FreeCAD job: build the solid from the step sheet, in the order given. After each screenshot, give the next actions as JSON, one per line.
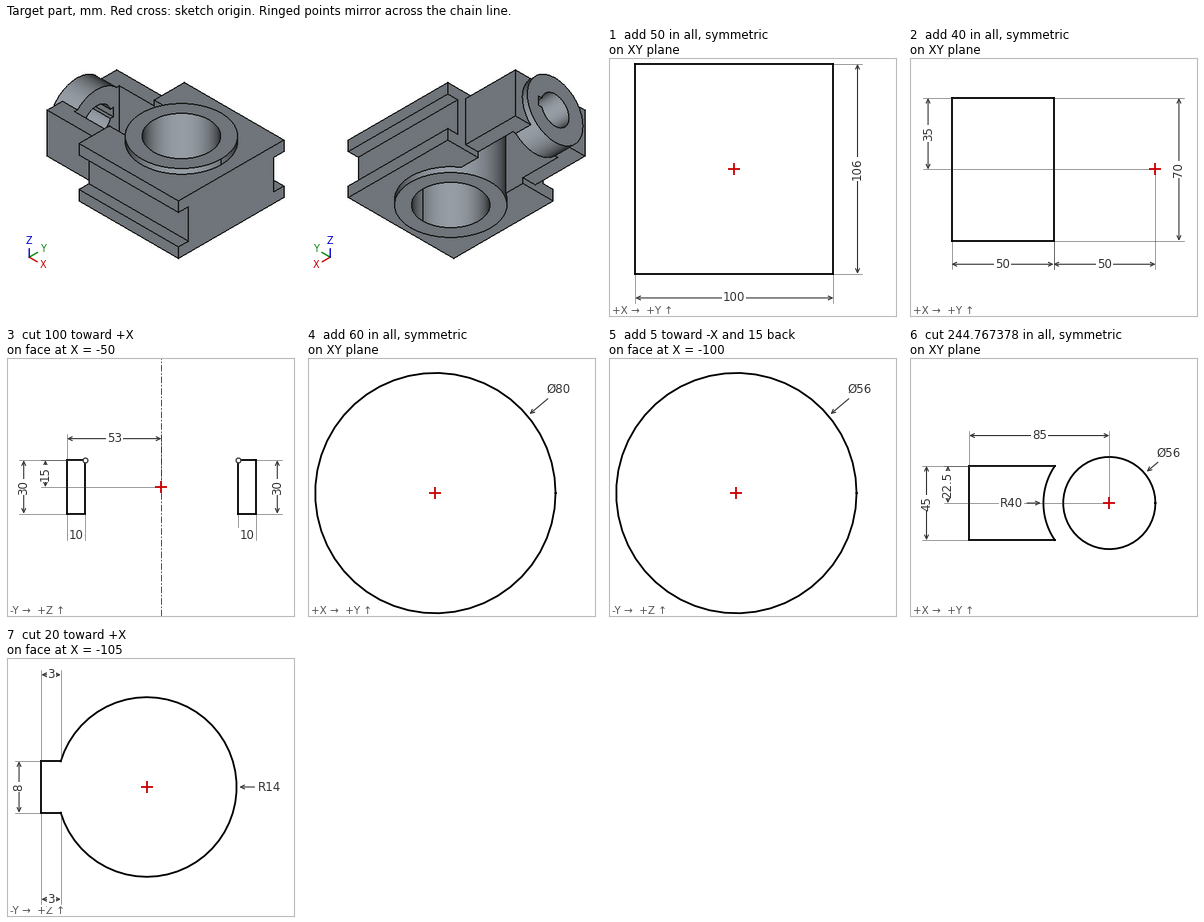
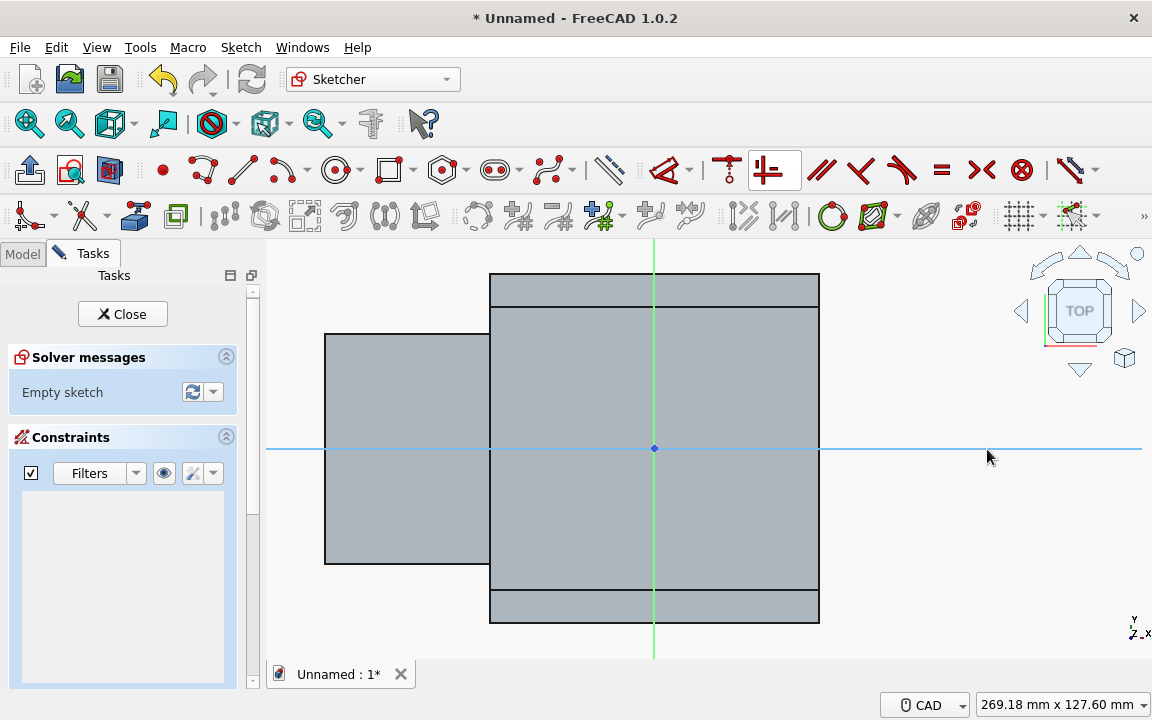
{"action": "left_click", "coordinate": [336, 170]}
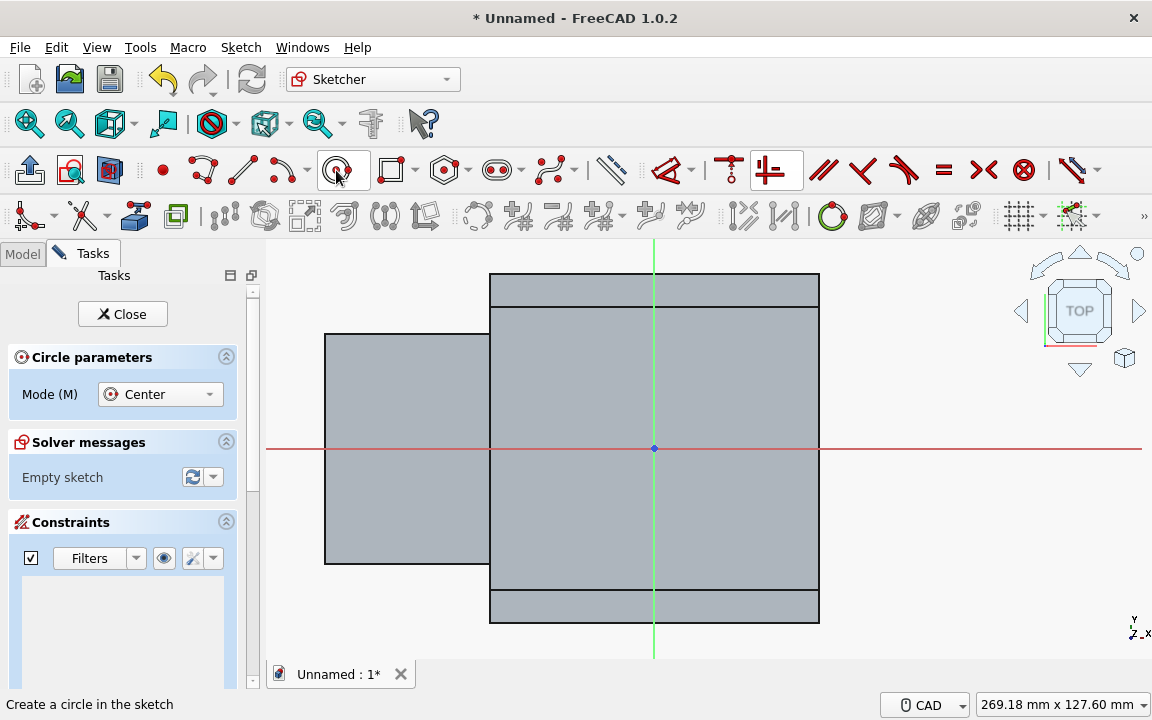
{"action": "left_click", "coordinate": [654, 449]}
{"action": "mouse_move", "coordinate": [747, 356]}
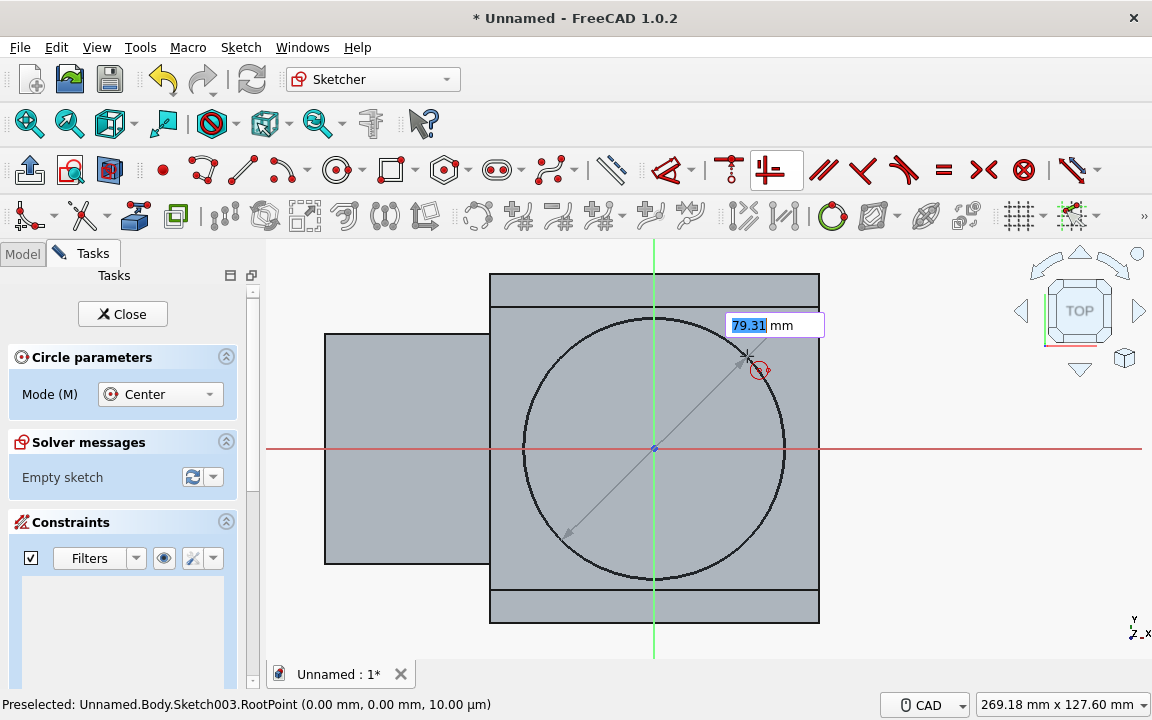
{"action": "type", "text": "80"}
{"action": "key", "text": "Return"}
{"action": "key", "text": "Escape"}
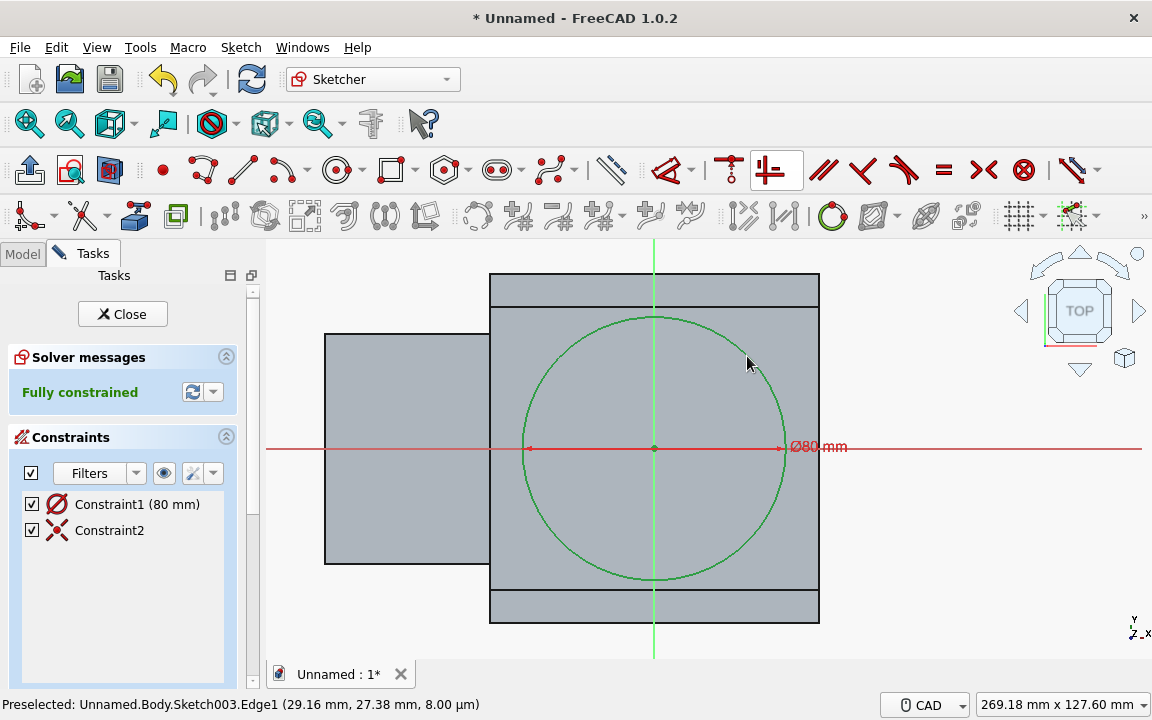
{"action": "left_click", "coordinate": [123, 314]}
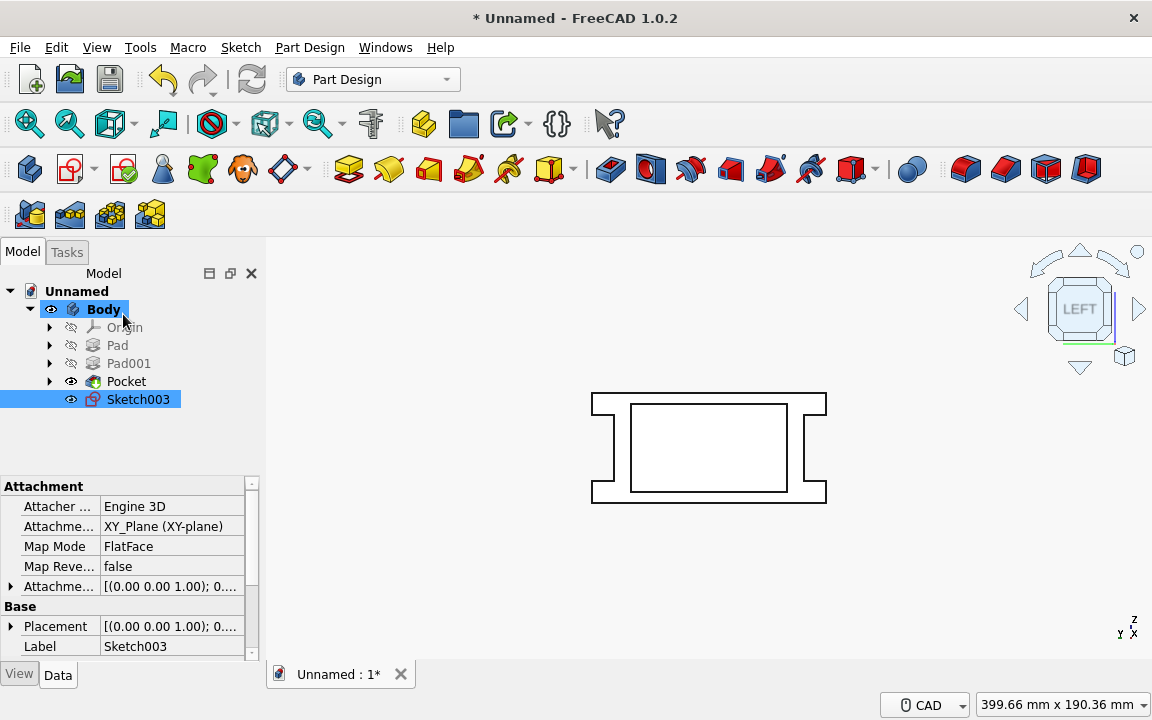
{"action": "left_click", "coordinate": [350, 170]}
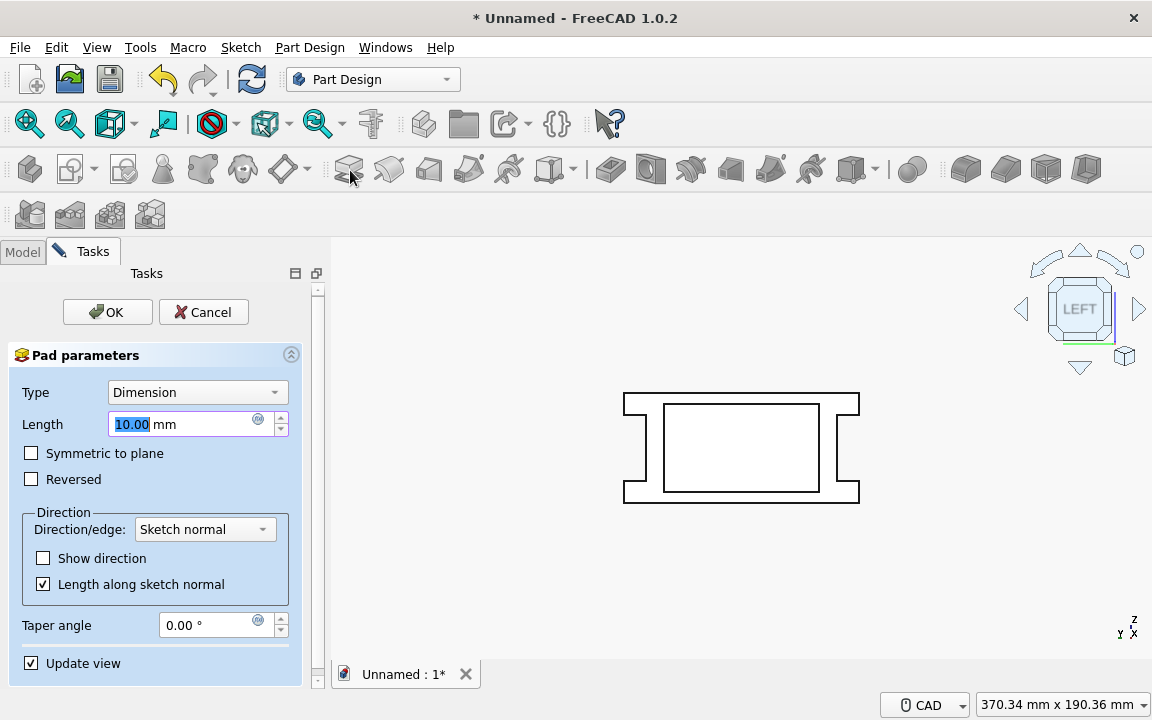
{"action": "type", "text": "60"}
{"action": "key", "text": "Tab"}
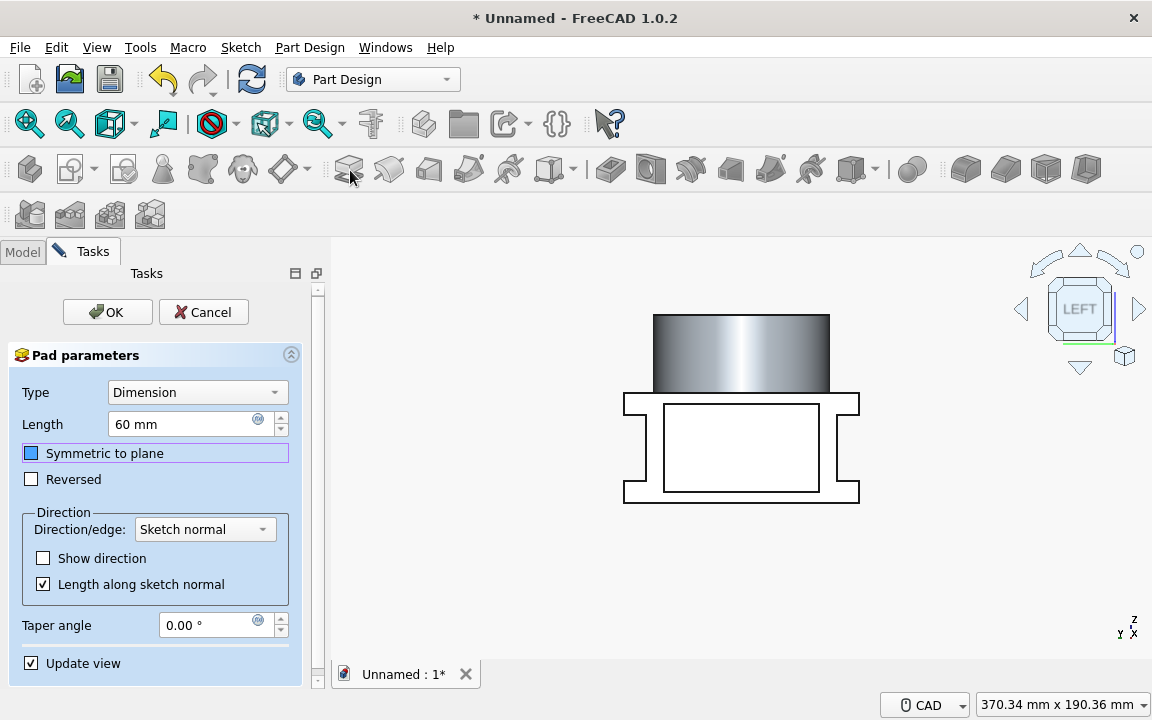
{"action": "left_click", "coordinate": [30, 453]}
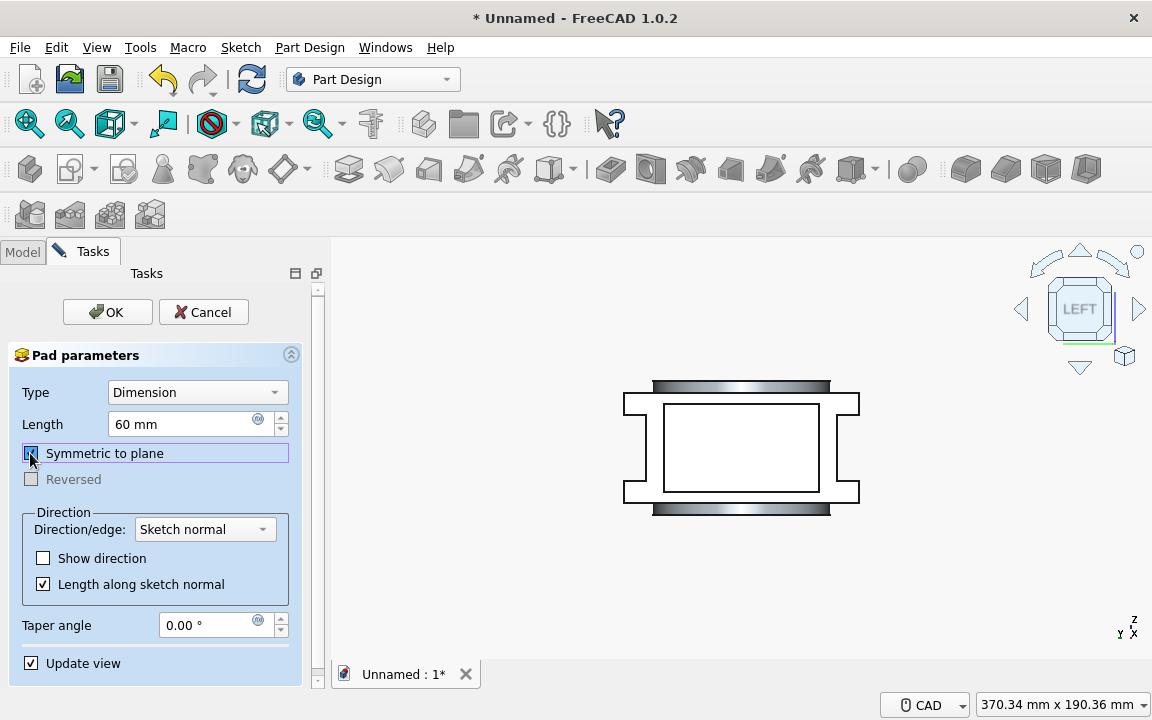
{"action": "left_click", "coordinate": [108, 312]}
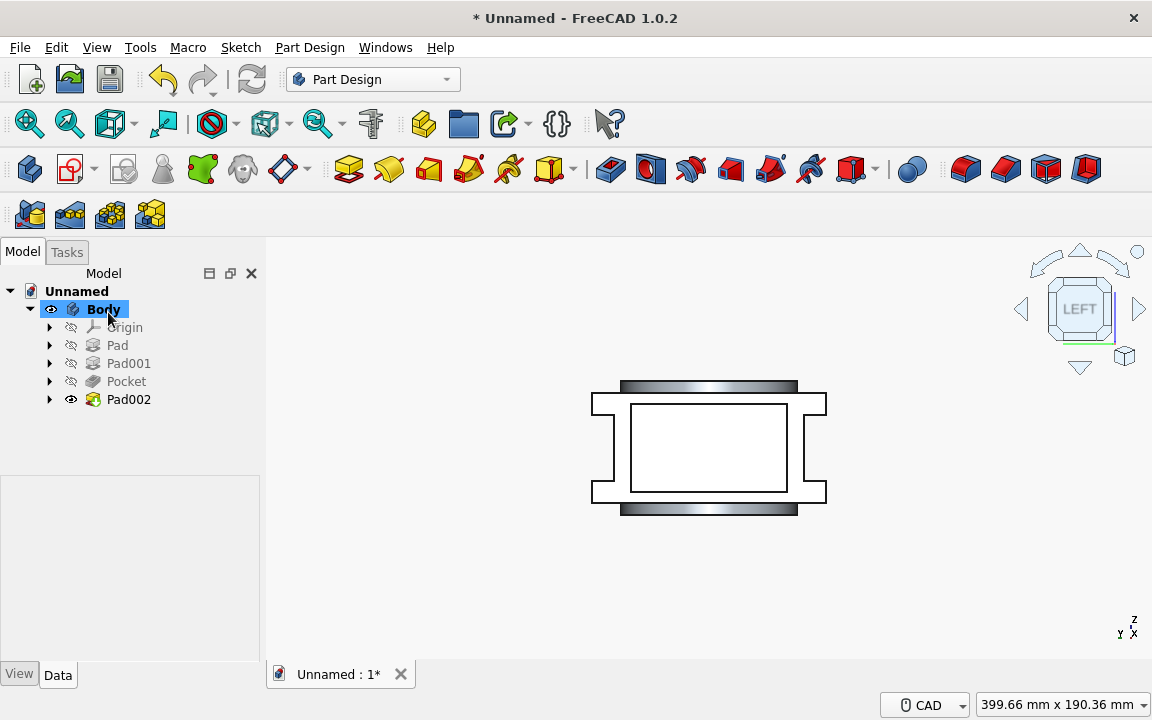
{"action": "left_click", "coordinate": [30, 124]}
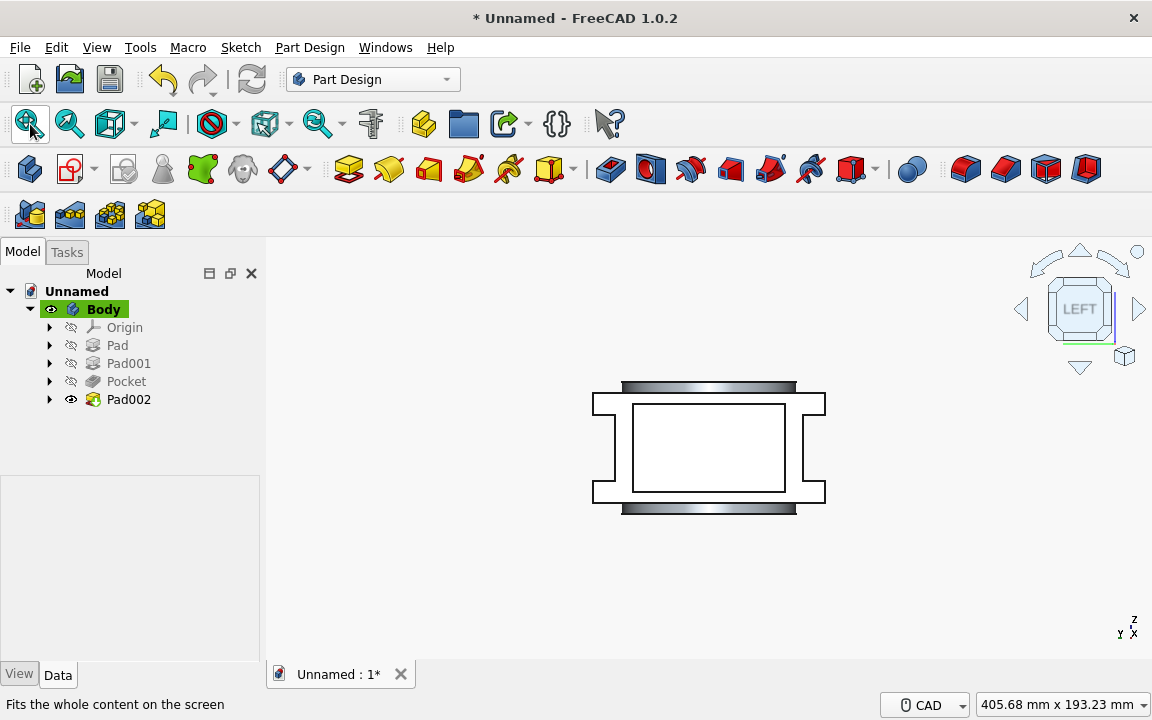
{"action": "left_click", "coordinate": [687, 447]}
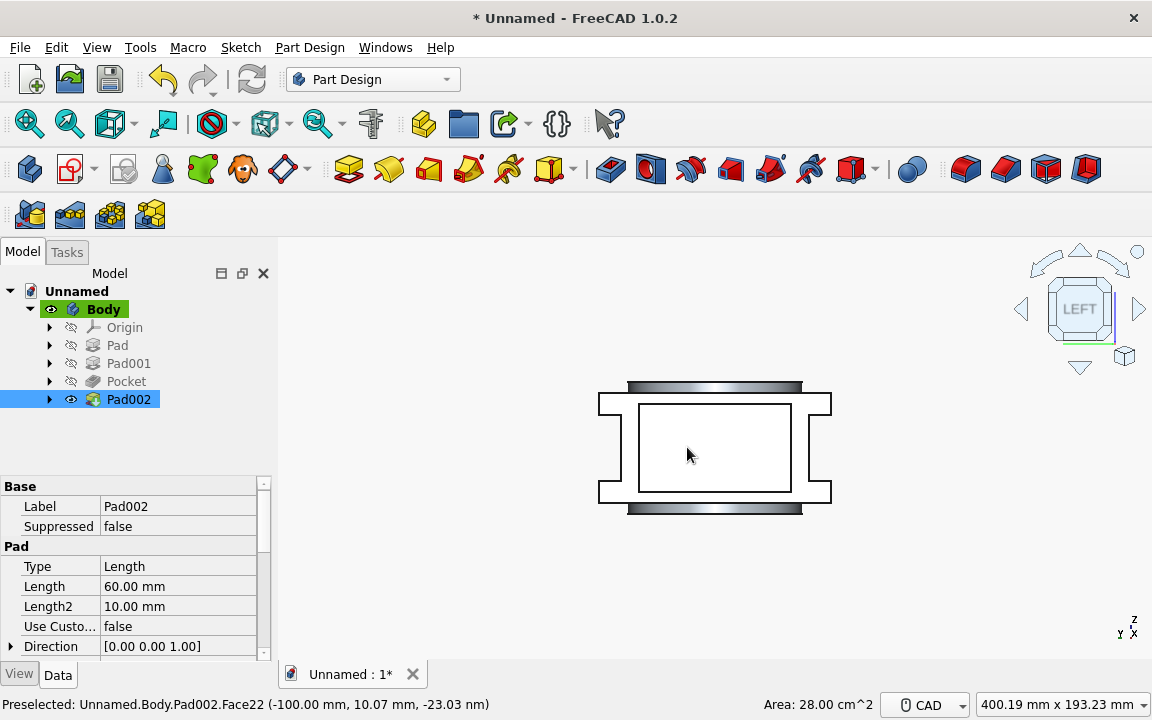
{"action": "left_click", "coordinate": [70, 170]}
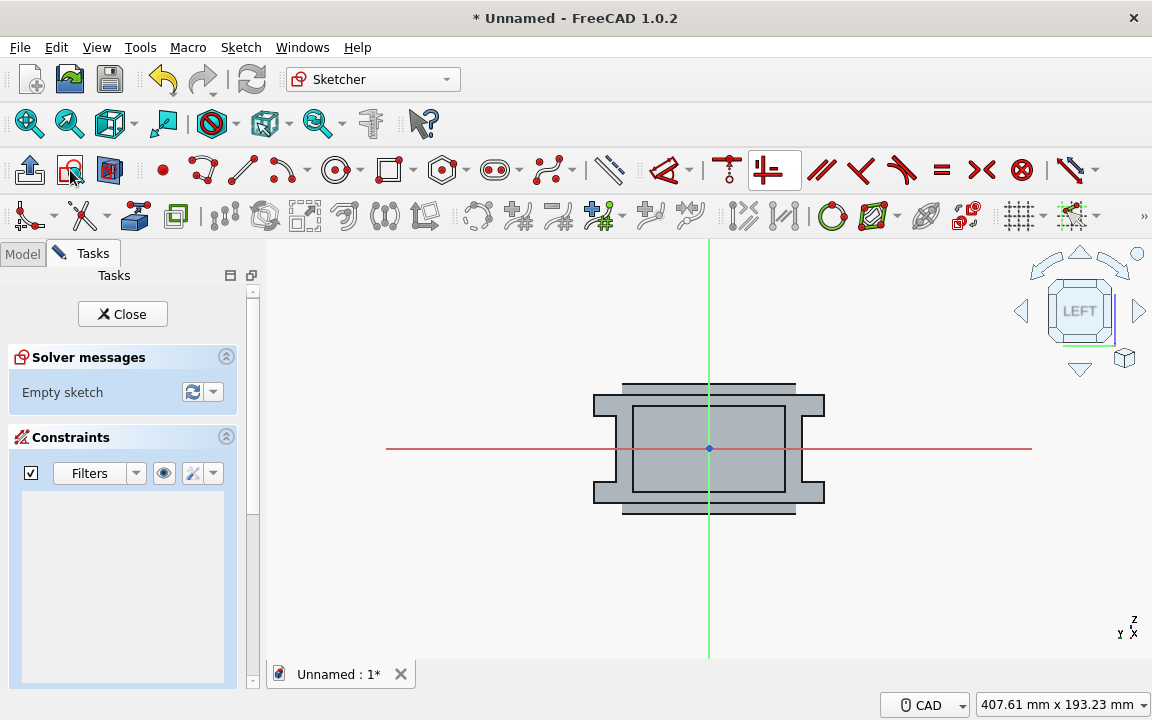
{"action": "scroll", "coordinate": [765, 449], "scroll_direction": "up", "scroll_amount": 4}